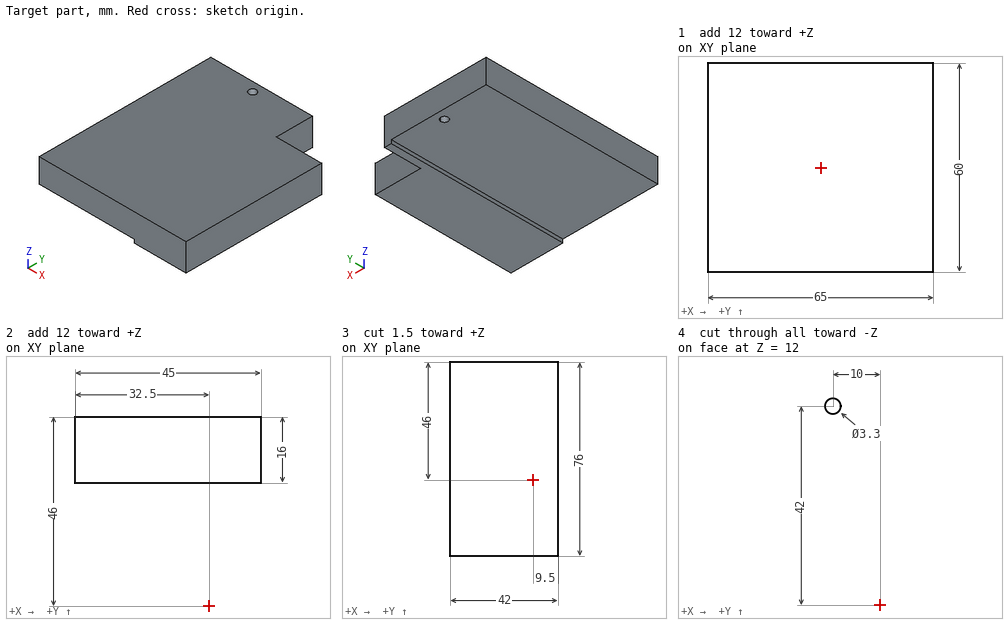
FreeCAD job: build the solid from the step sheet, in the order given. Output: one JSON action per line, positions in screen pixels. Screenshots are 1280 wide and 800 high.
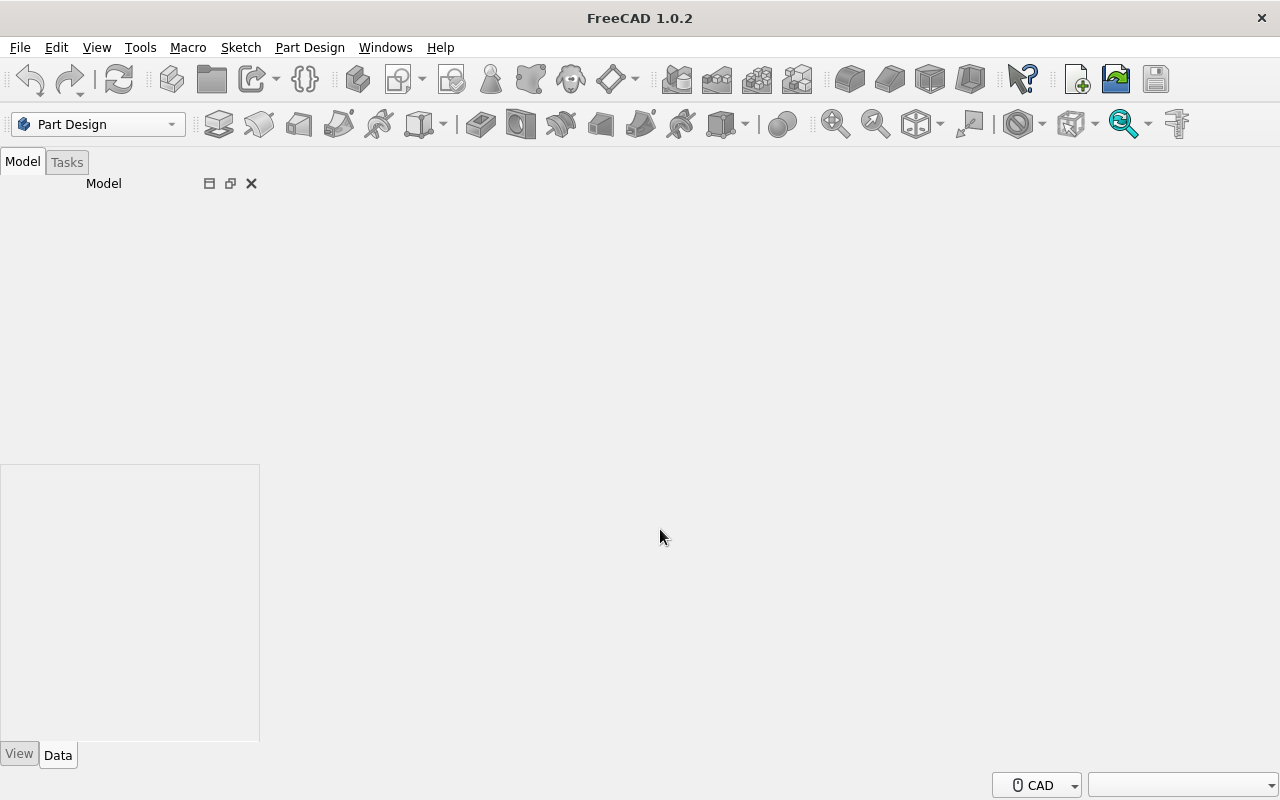
{"action": "left_click", "coordinate": [1076, 80]}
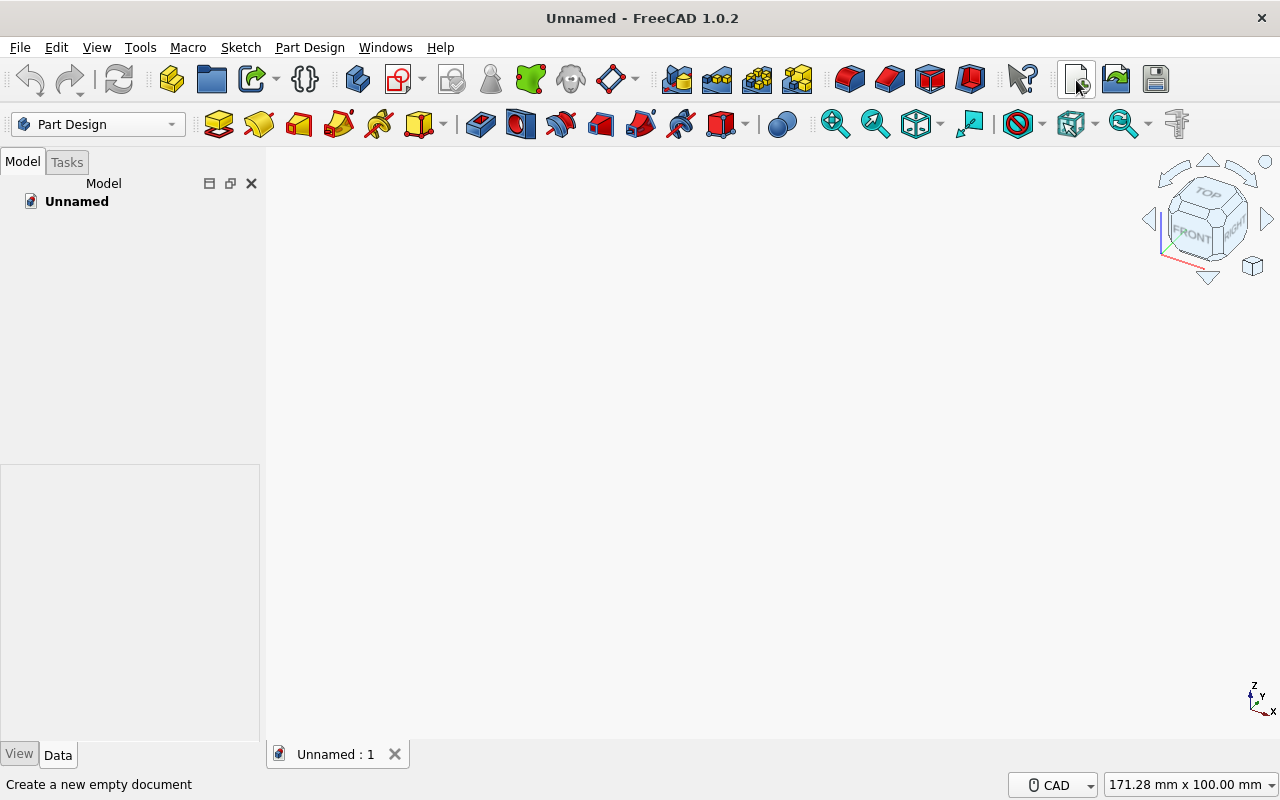
{"action": "left_click", "coordinate": [398, 80]}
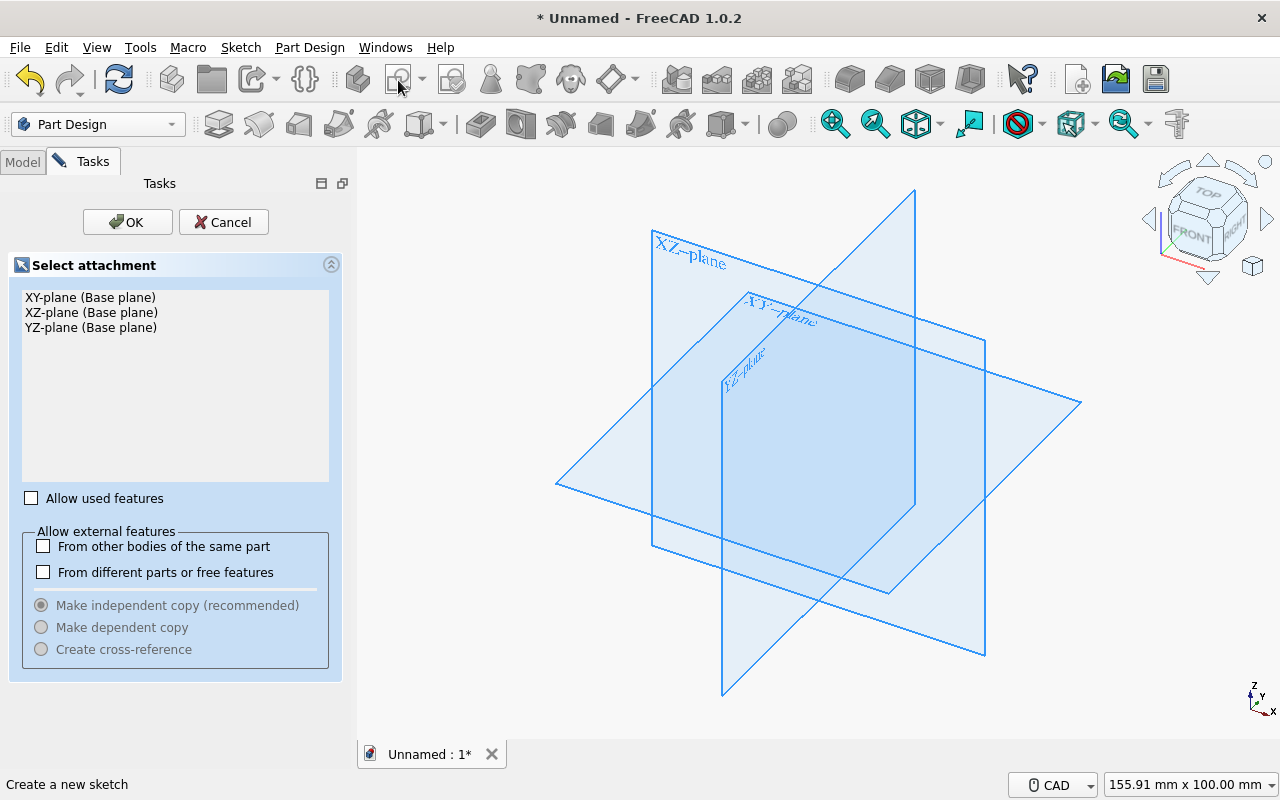
{"action": "left_click", "coordinate": [82, 298]}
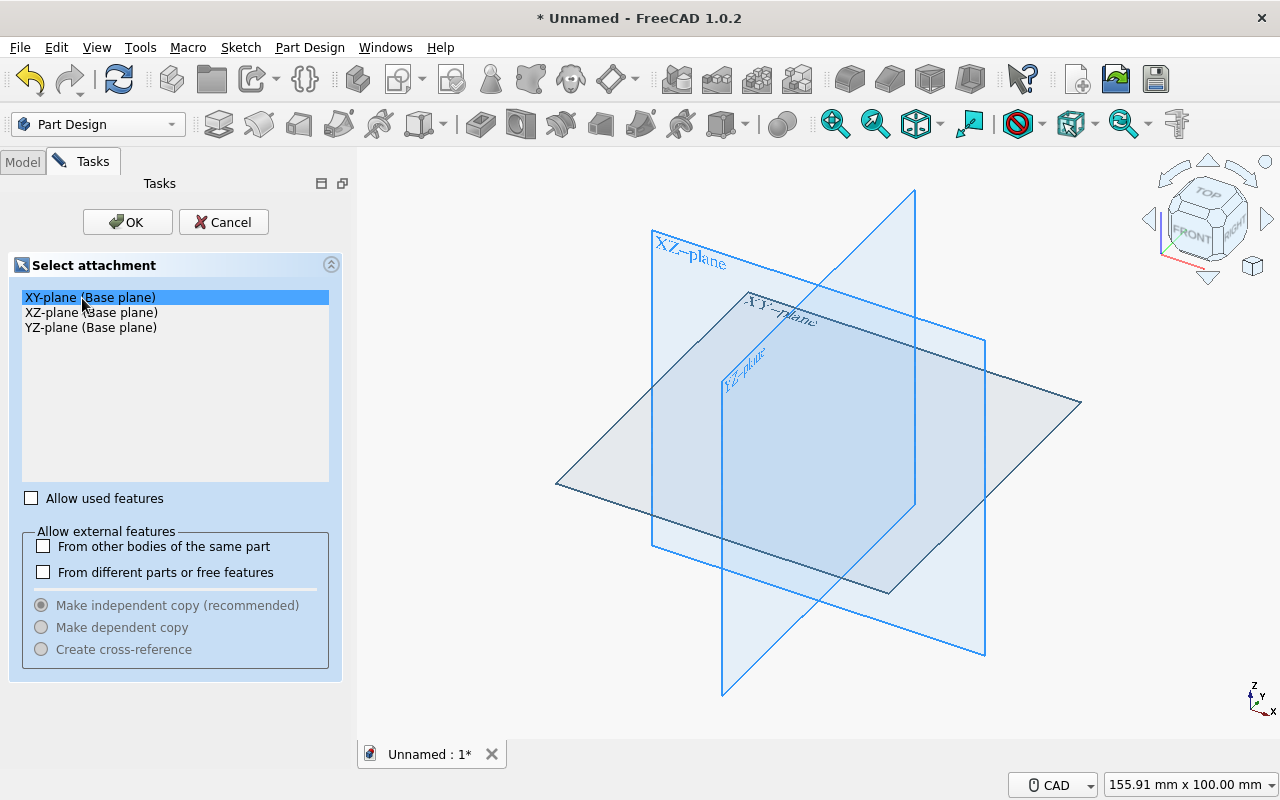
{"action": "left_click", "coordinate": [128, 222]}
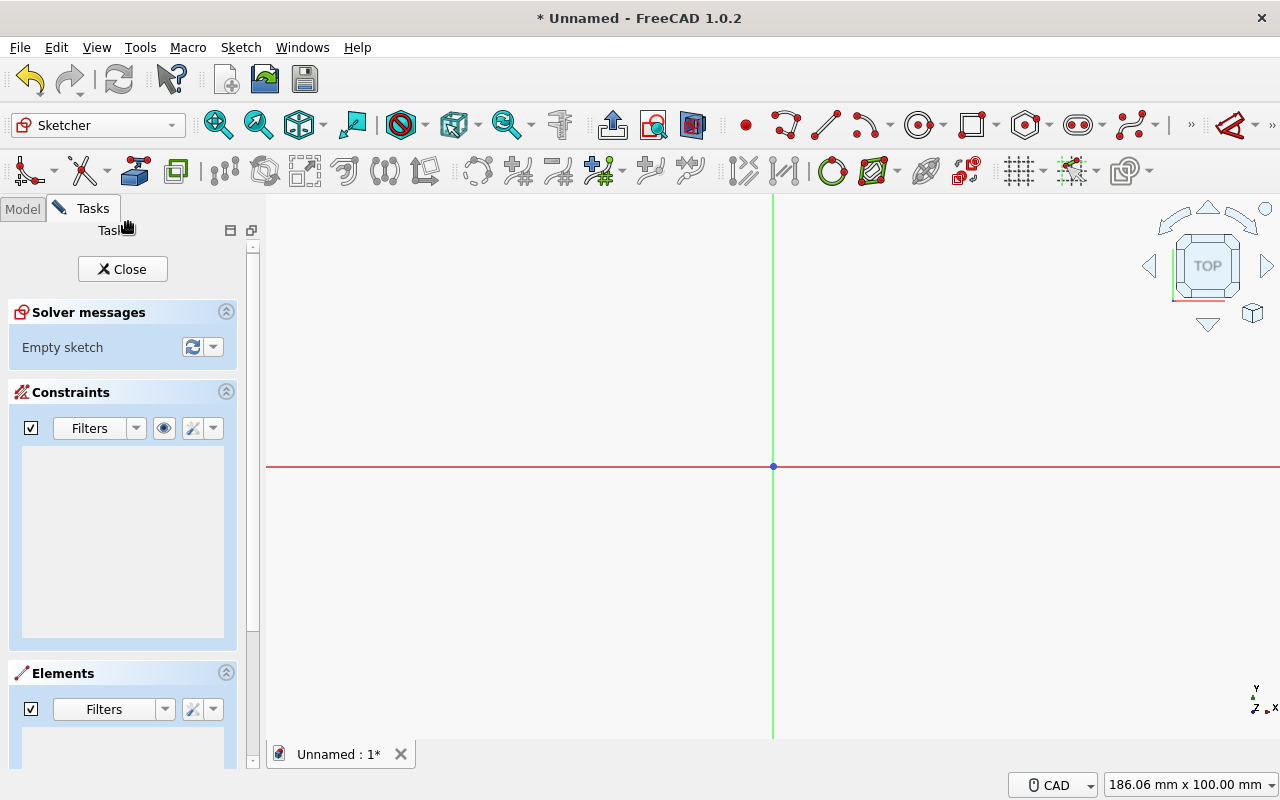
{"action": "left_click", "coordinate": [998, 126]}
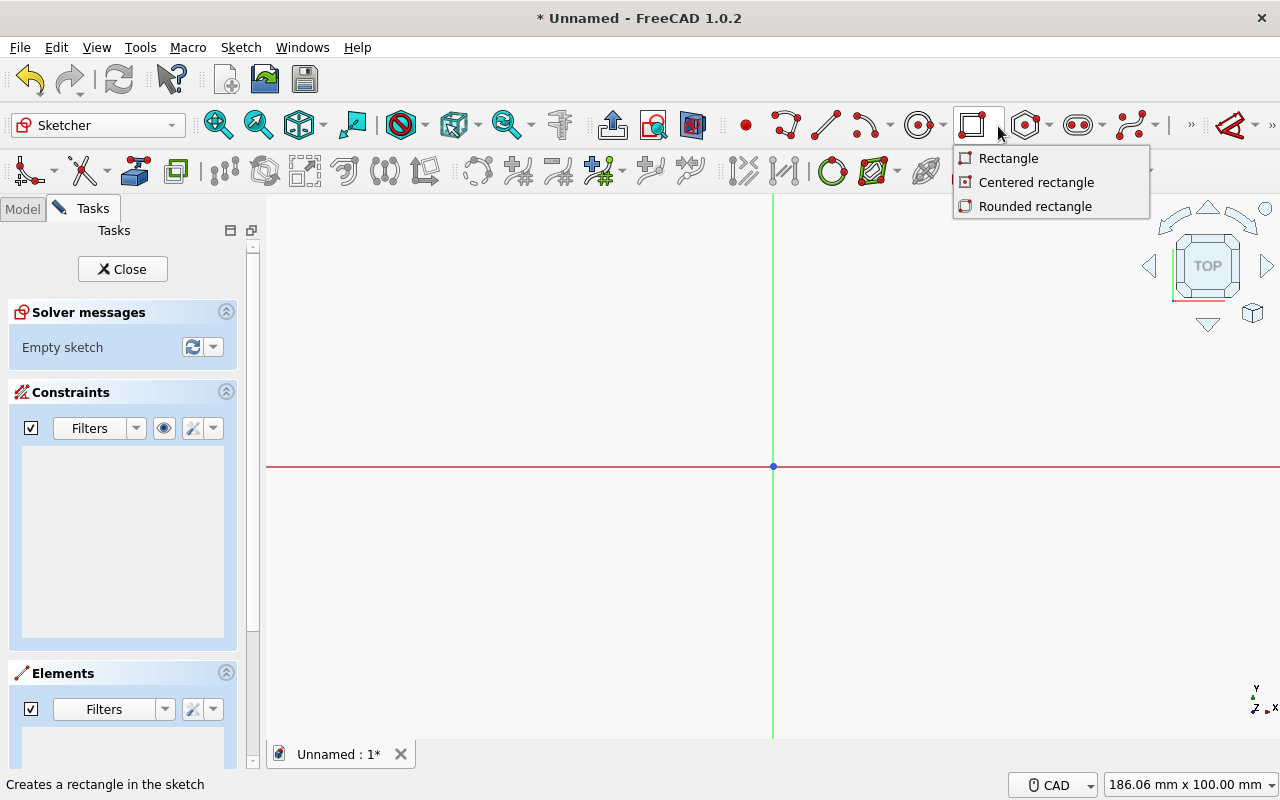
{"action": "left_click", "coordinate": [1052, 182]}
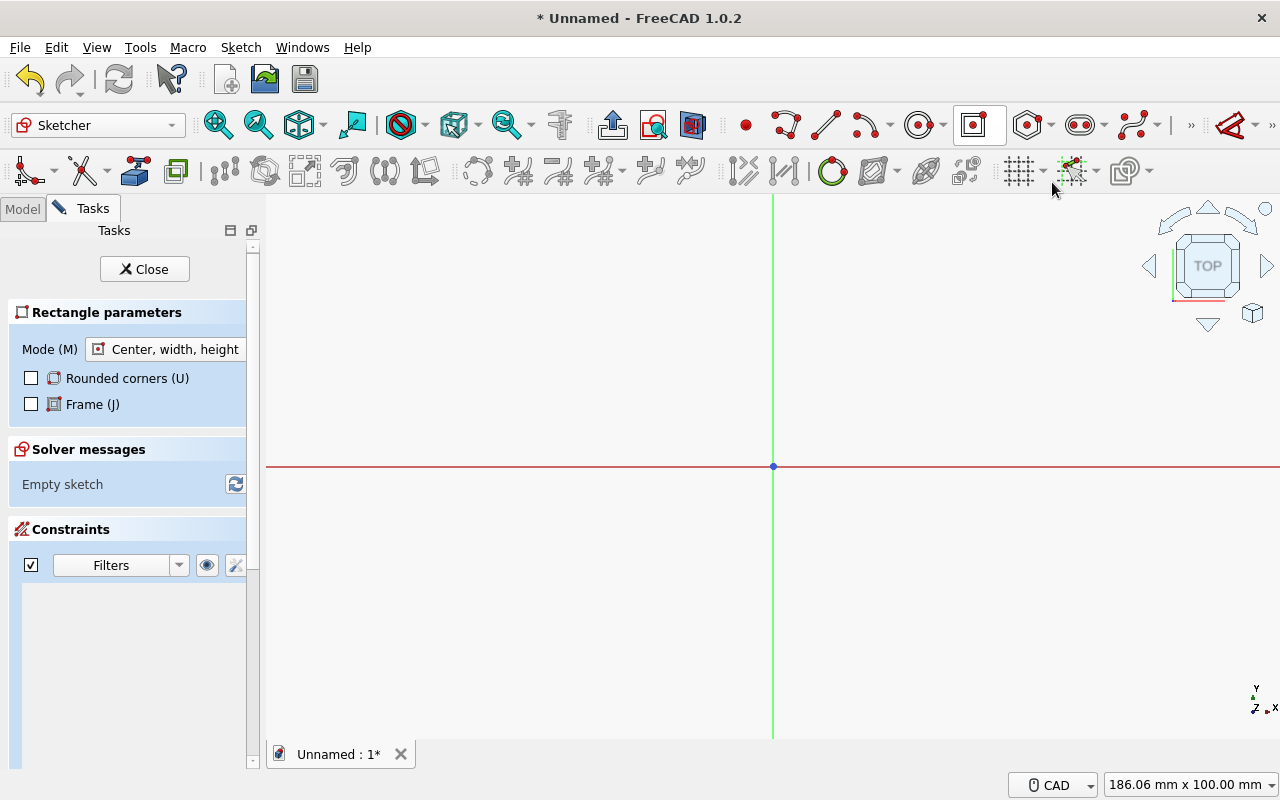
{"action": "left_click", "coordinate": [773, 466]}
{"action": "mouse_move", "coordinate": [950, 303]}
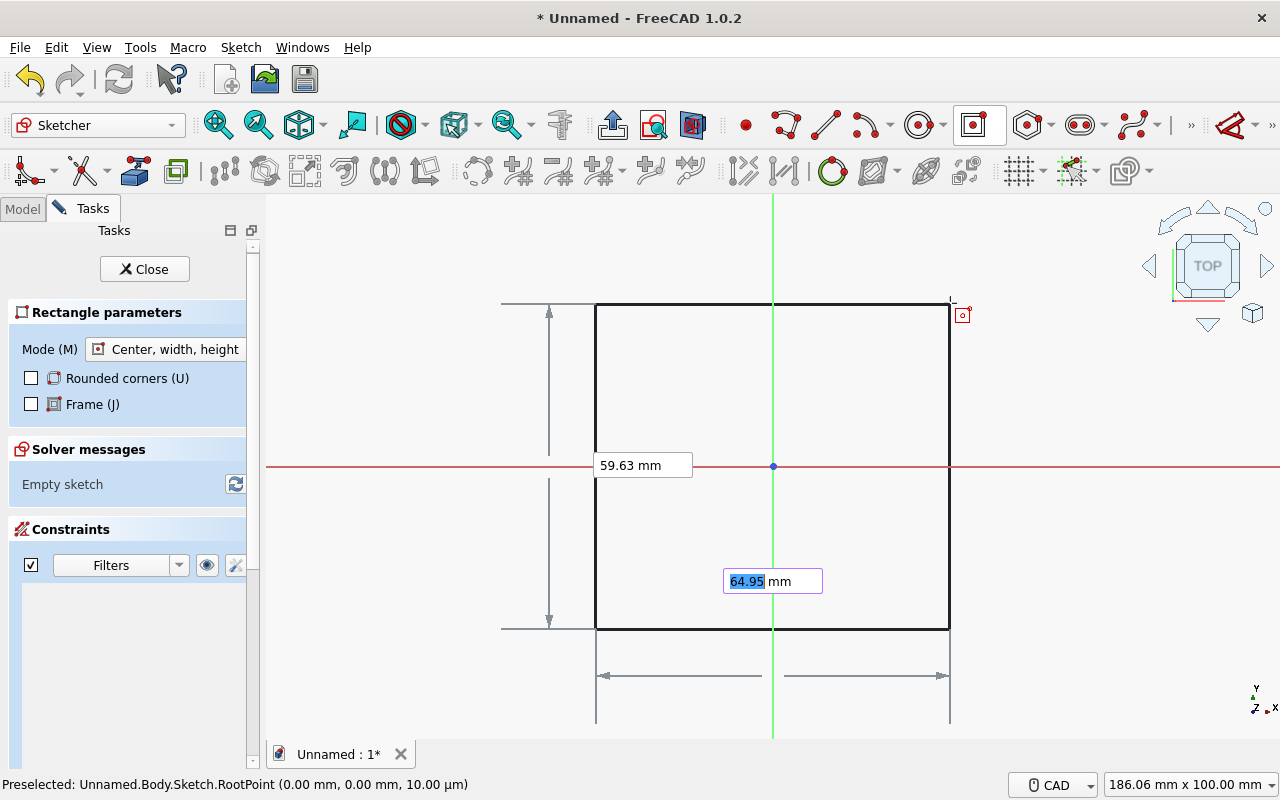
{"action": "type", "text": "65"}
{"action": "key", "text": "Tab"}
{"action": "type", "text": "60"}
{"action": "key", "text": "Return"}
{"action": "key", "text": "Escape"}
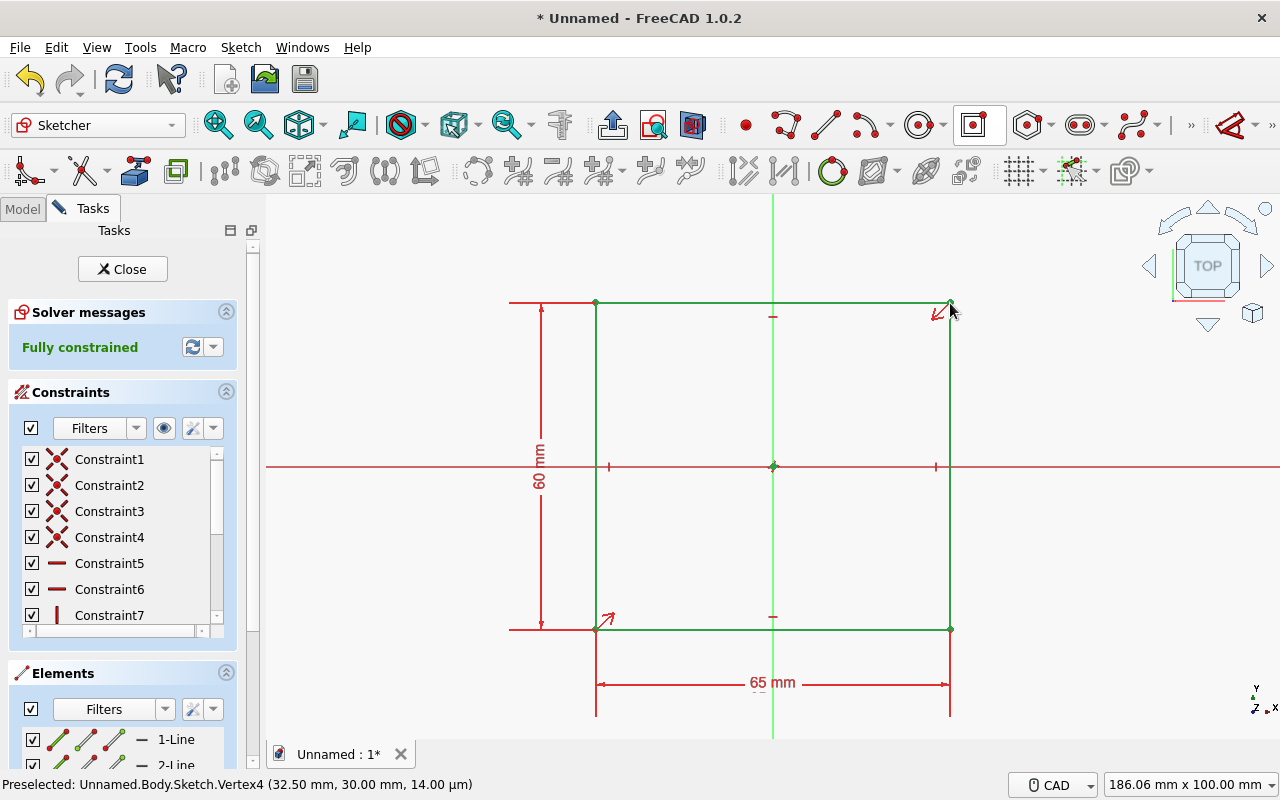
{"action": "left_click", "coordinate": [123, 269]}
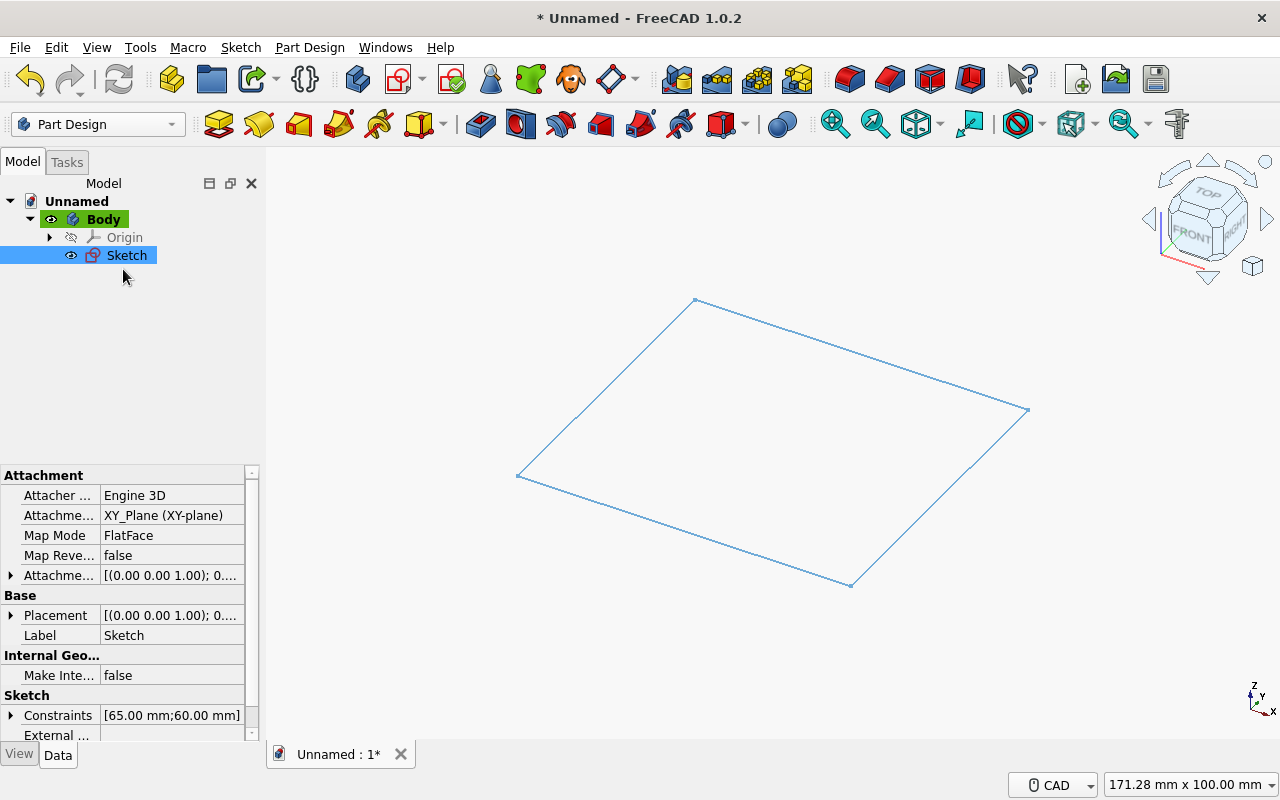
{"action": "left_click", "coordinate": [220, 124]}